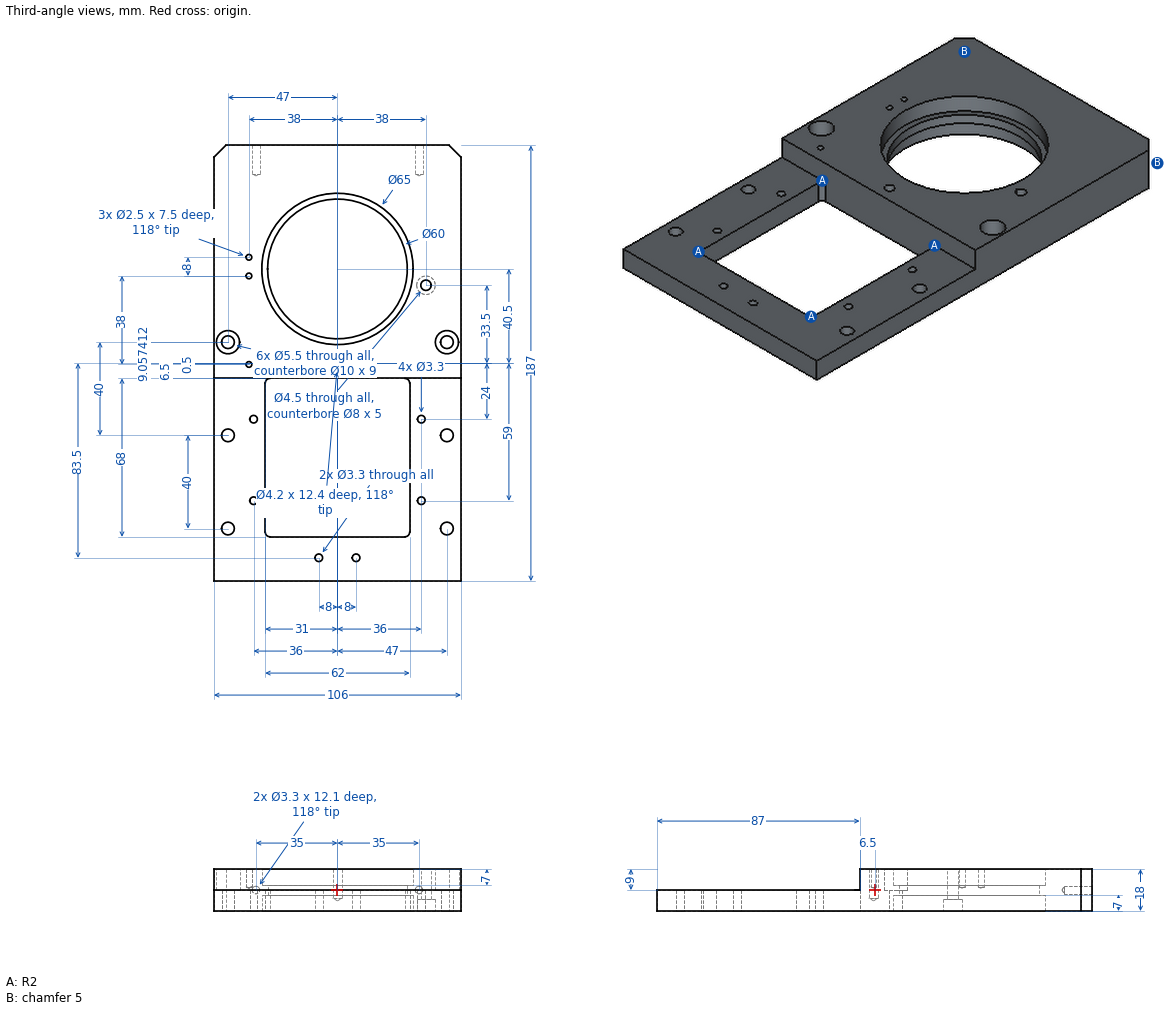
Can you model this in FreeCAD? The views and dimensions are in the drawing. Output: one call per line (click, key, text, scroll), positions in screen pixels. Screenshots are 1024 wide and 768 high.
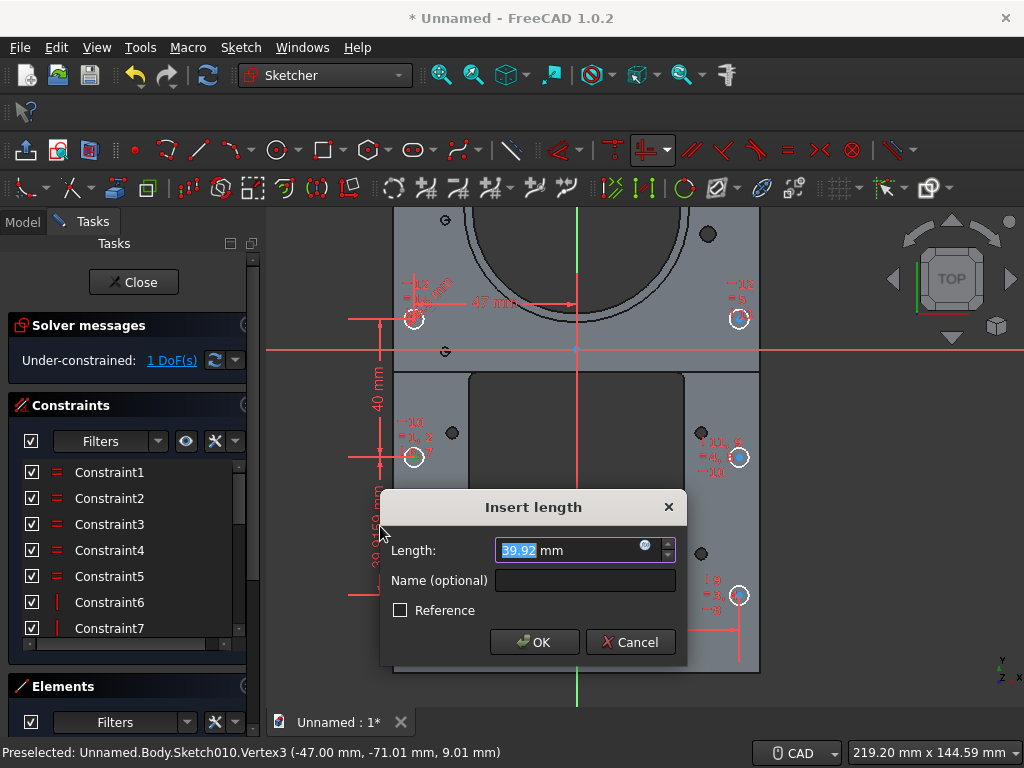
text(40)
key(Return)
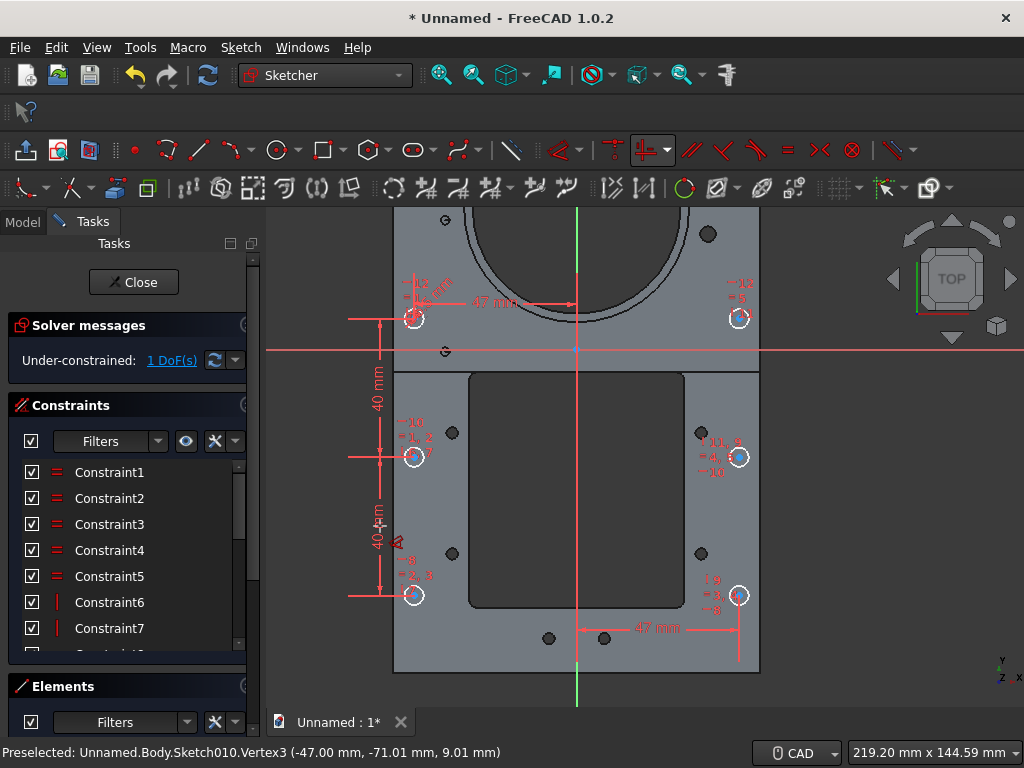
scroll(414, 319, up, 2)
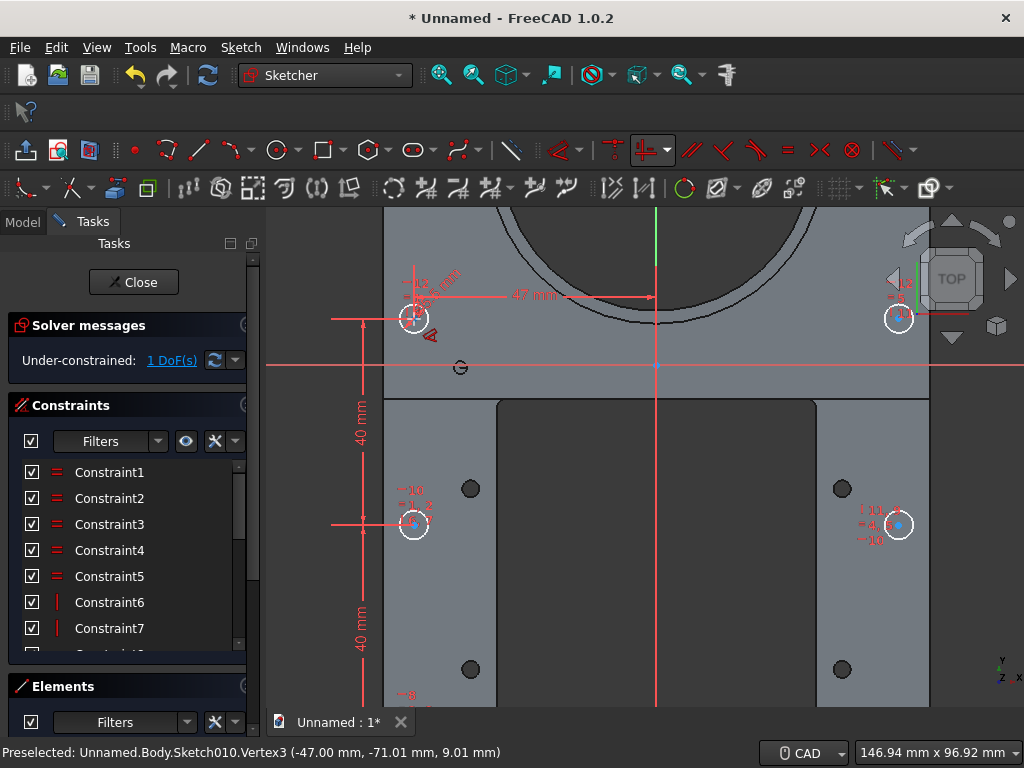
click(414, 319)
click(380, 342)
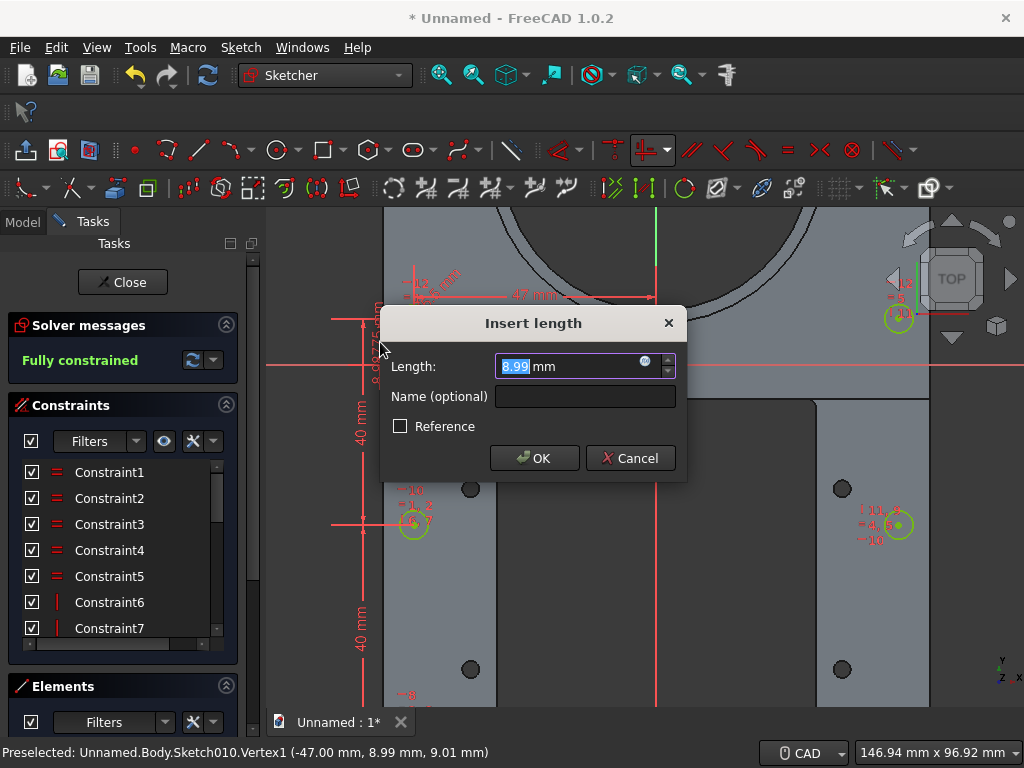
text(9.057412)
key(Return)
key(Escape)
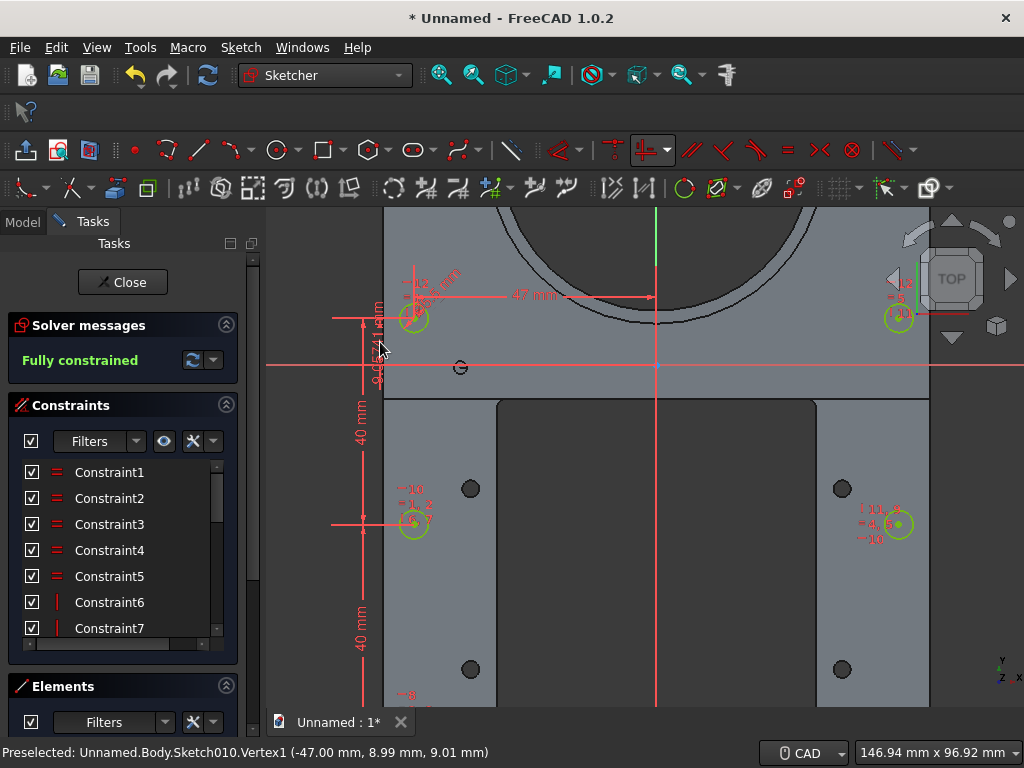
click(123, 282)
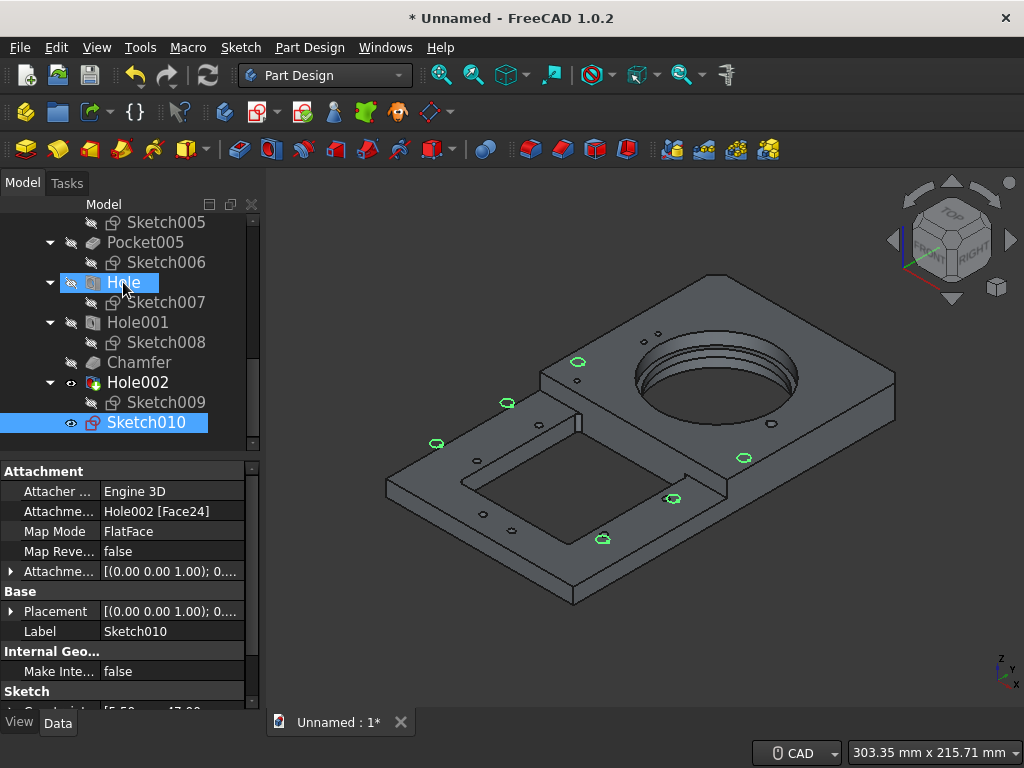
click(272, 150)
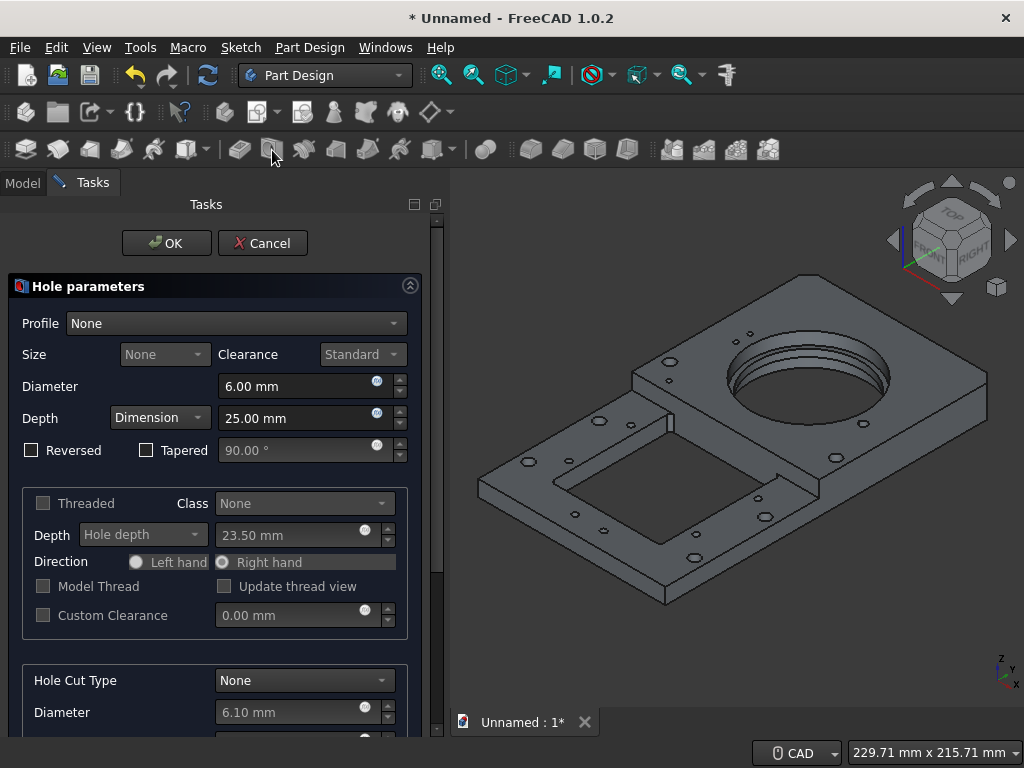
triple_click(305, 386)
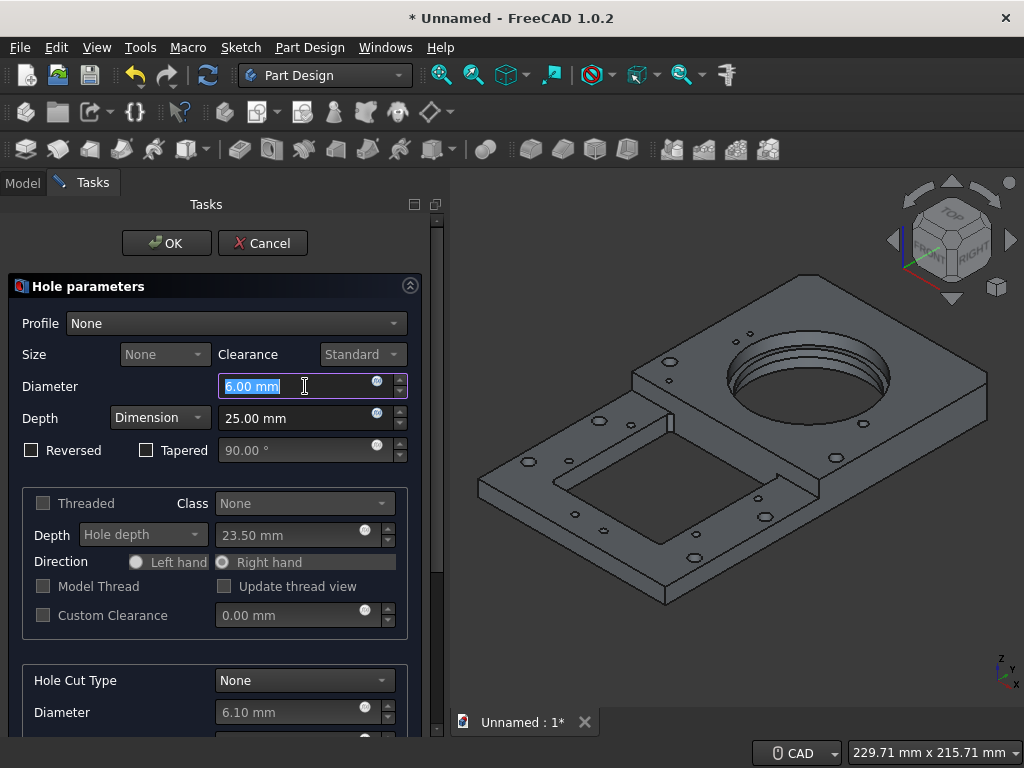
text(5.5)
key(Tab)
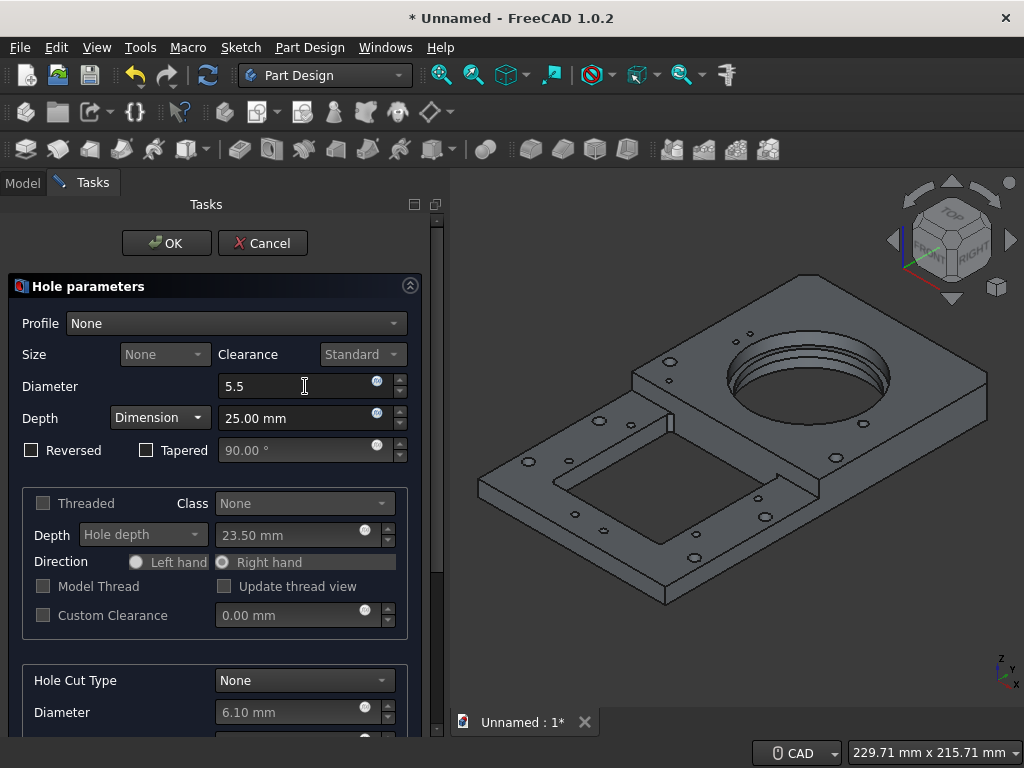
click(161, 418)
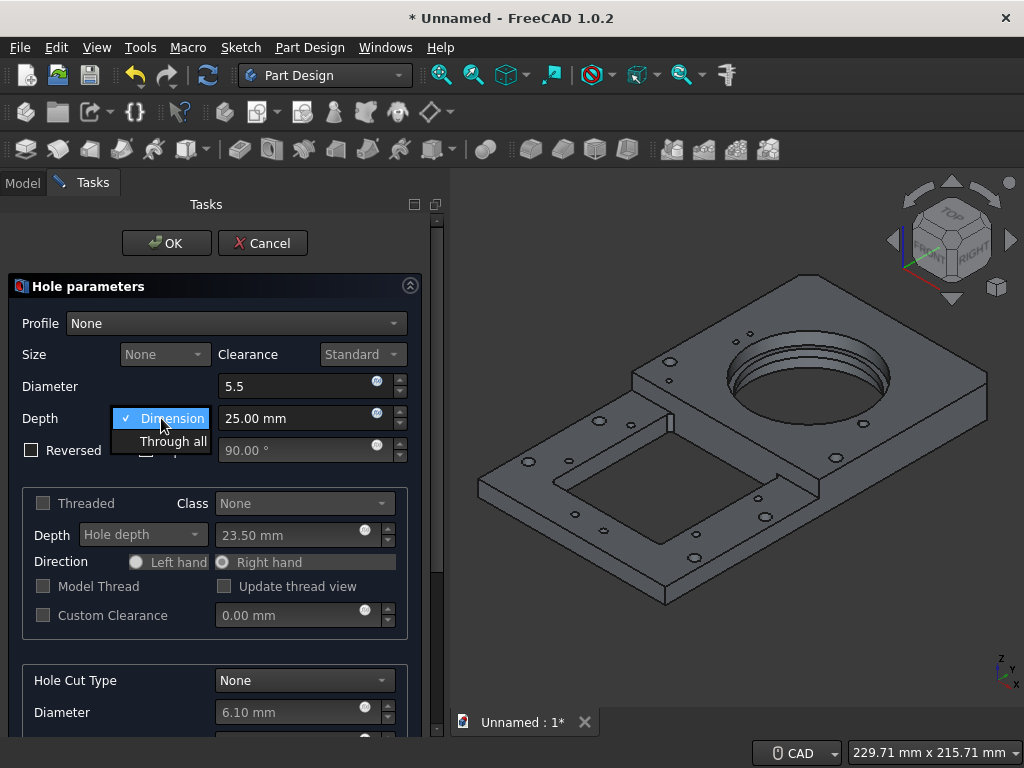
click(160, 442)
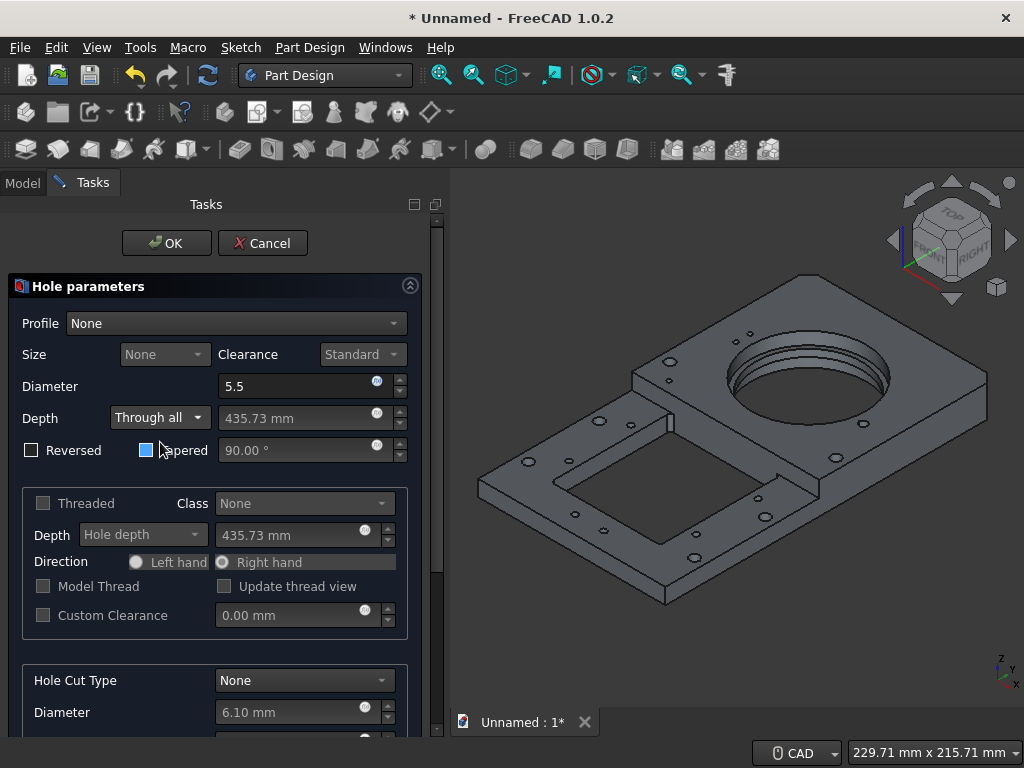
click(306, 680)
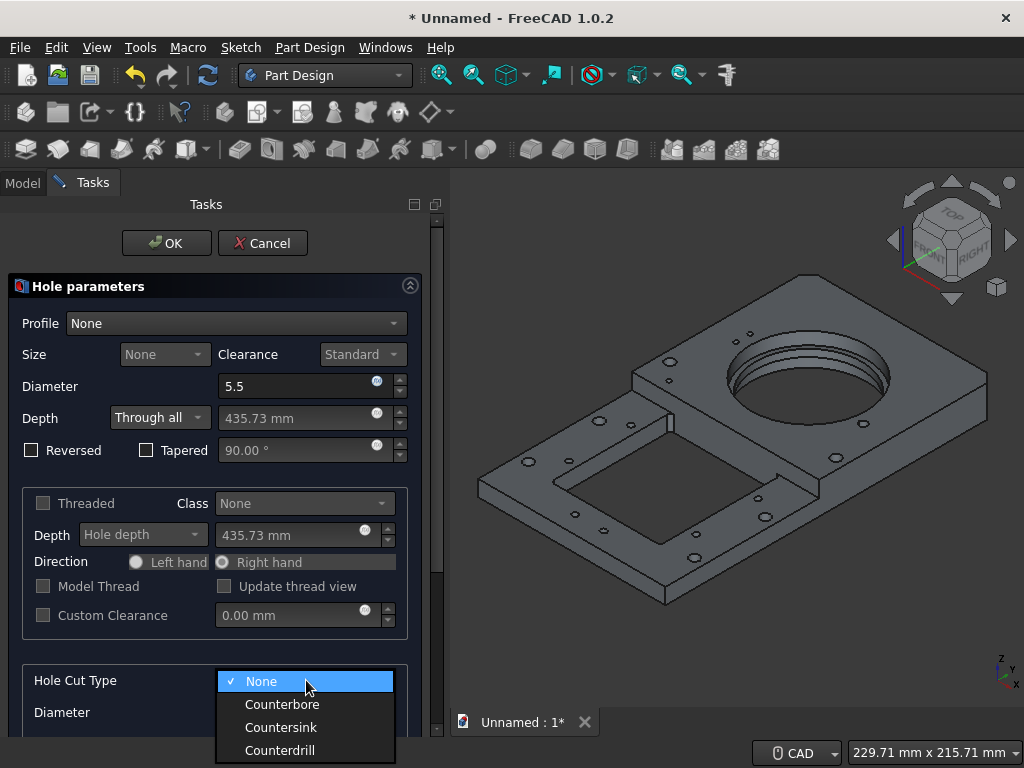
click(304, 704)